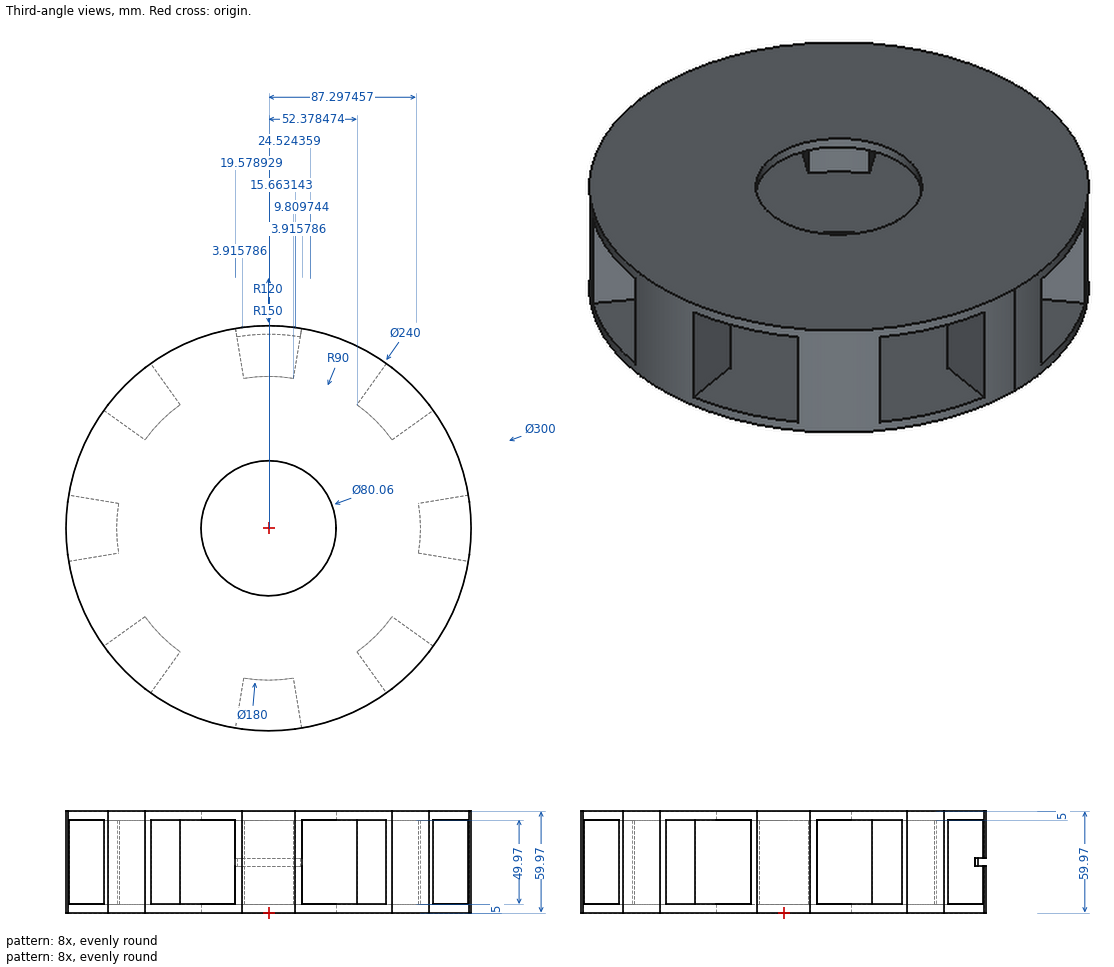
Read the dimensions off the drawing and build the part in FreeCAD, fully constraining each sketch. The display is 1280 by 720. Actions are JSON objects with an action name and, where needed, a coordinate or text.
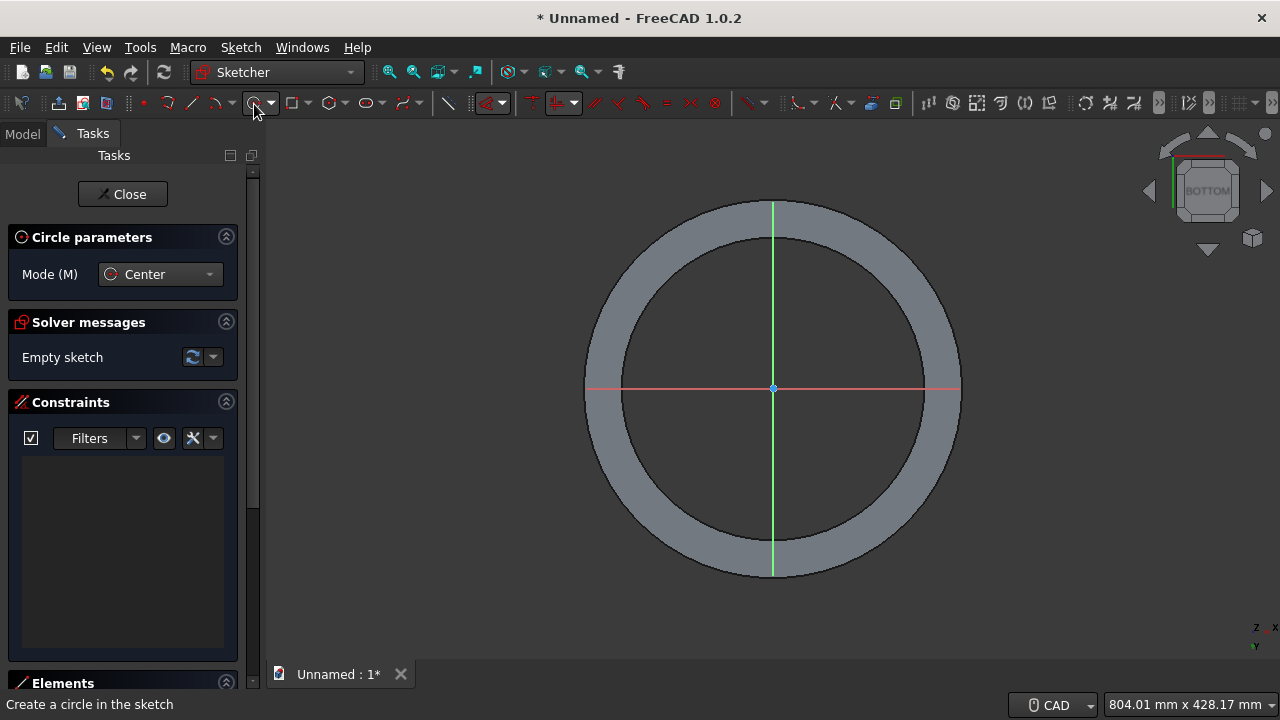
{"action": "left_click", "coordinate": [773, 389]}
{"action": "left_click", "coordinate": [880, 282]}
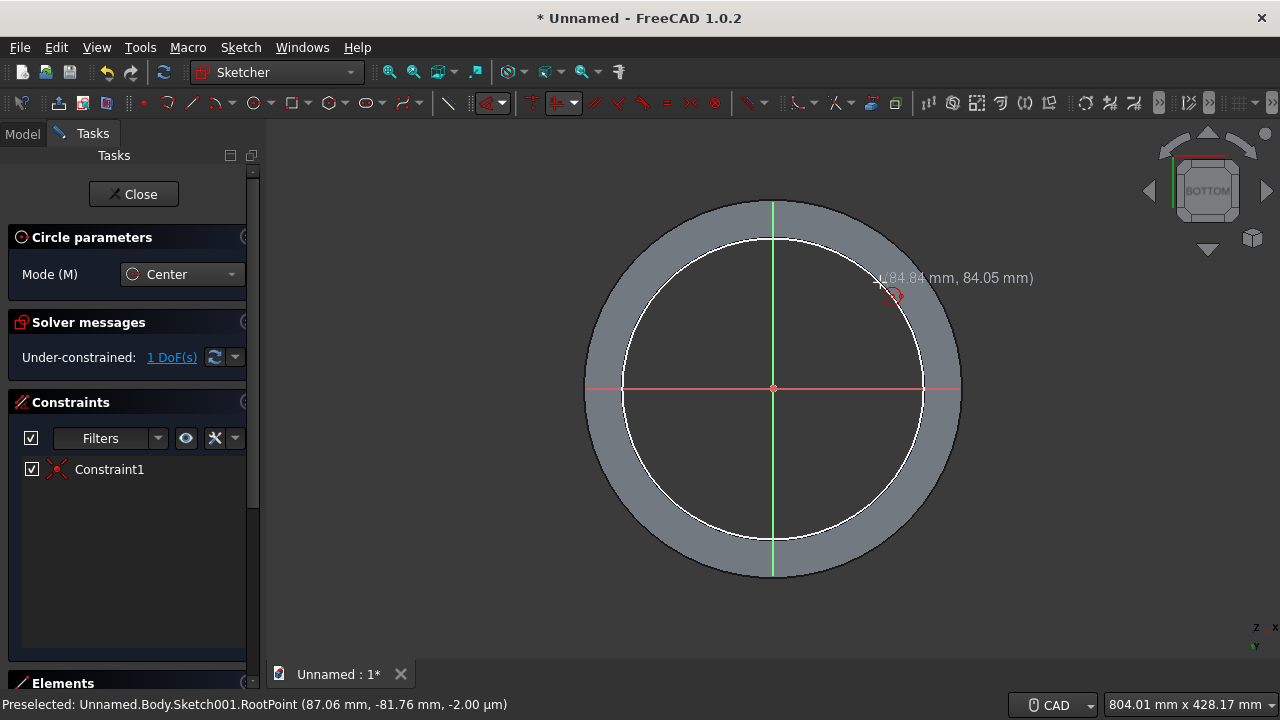
{"action": "left_click", "coordinate": [773, 389]}
{"action": "left_click", "coordinate": [853, 309]}
{"action": "key", "text": "Escape"}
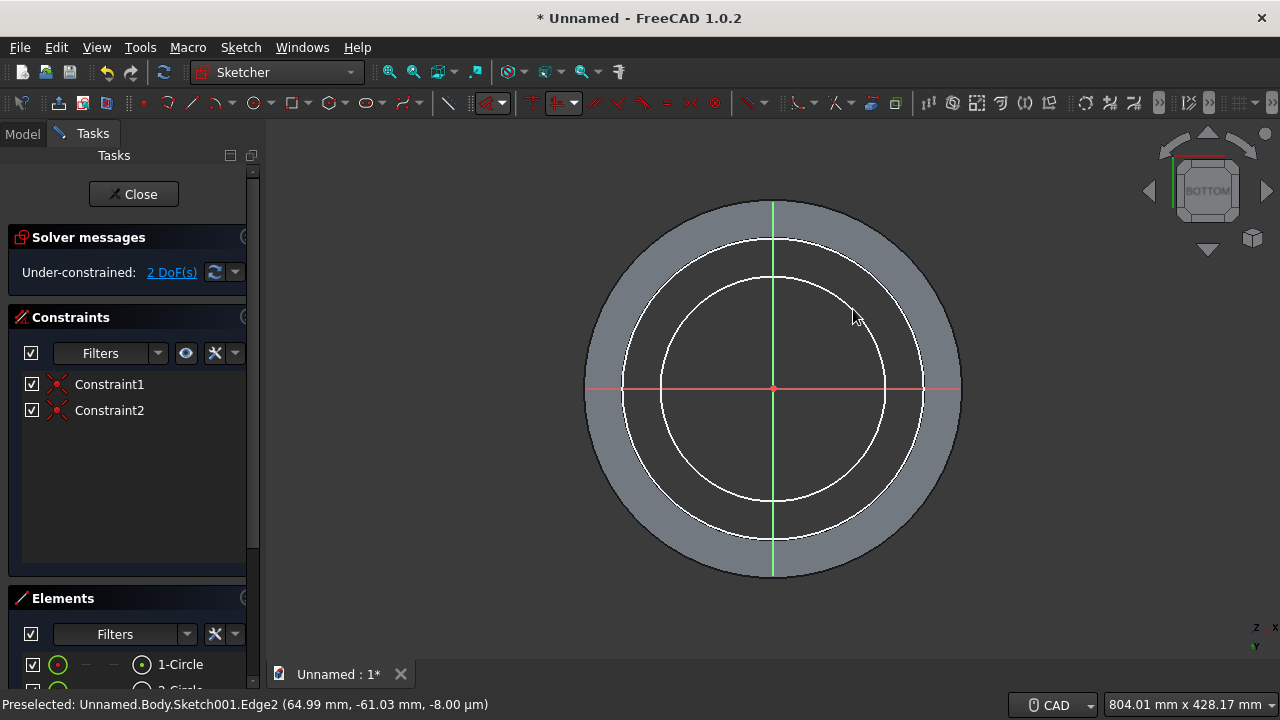
{"action": "left_click", "coordinate": [486, 104]}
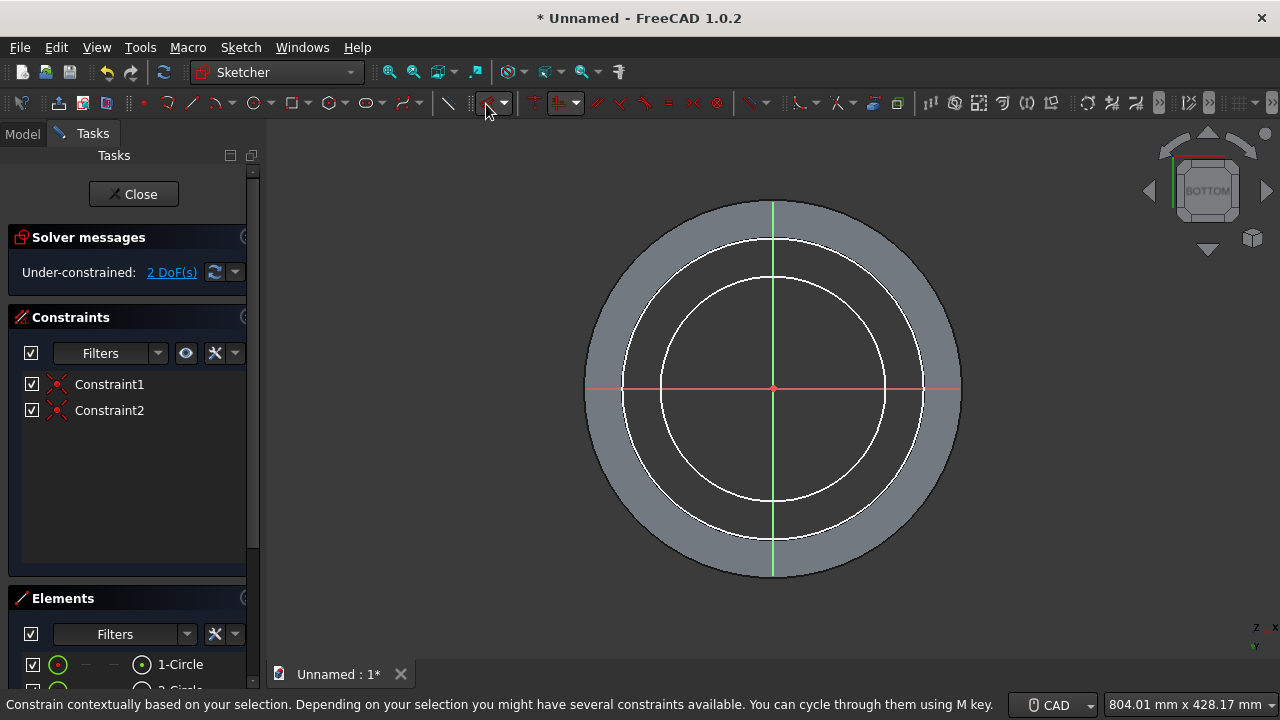
{"action": "left_click", "coordinate": [879, 282]}
{"action": "left_click", "coordinate": [902, 259]}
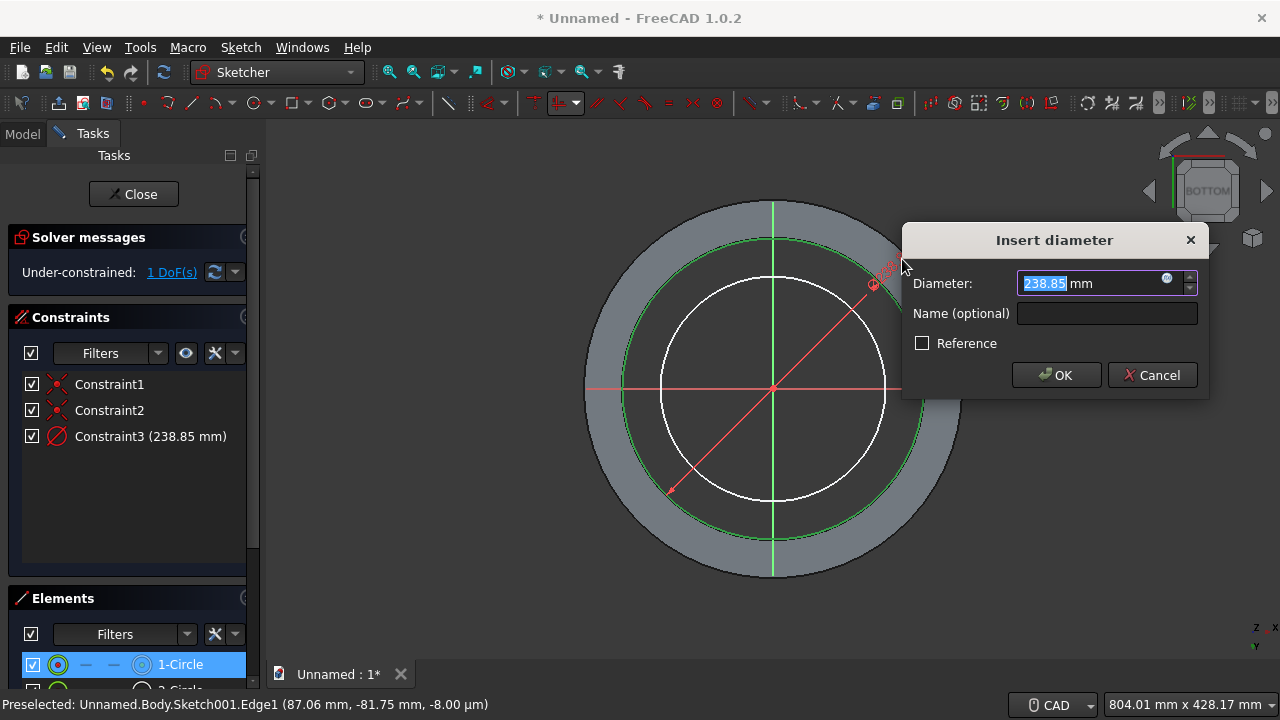
{"action": "type", "text": "240"}
{"action": "key", "text": "Return"}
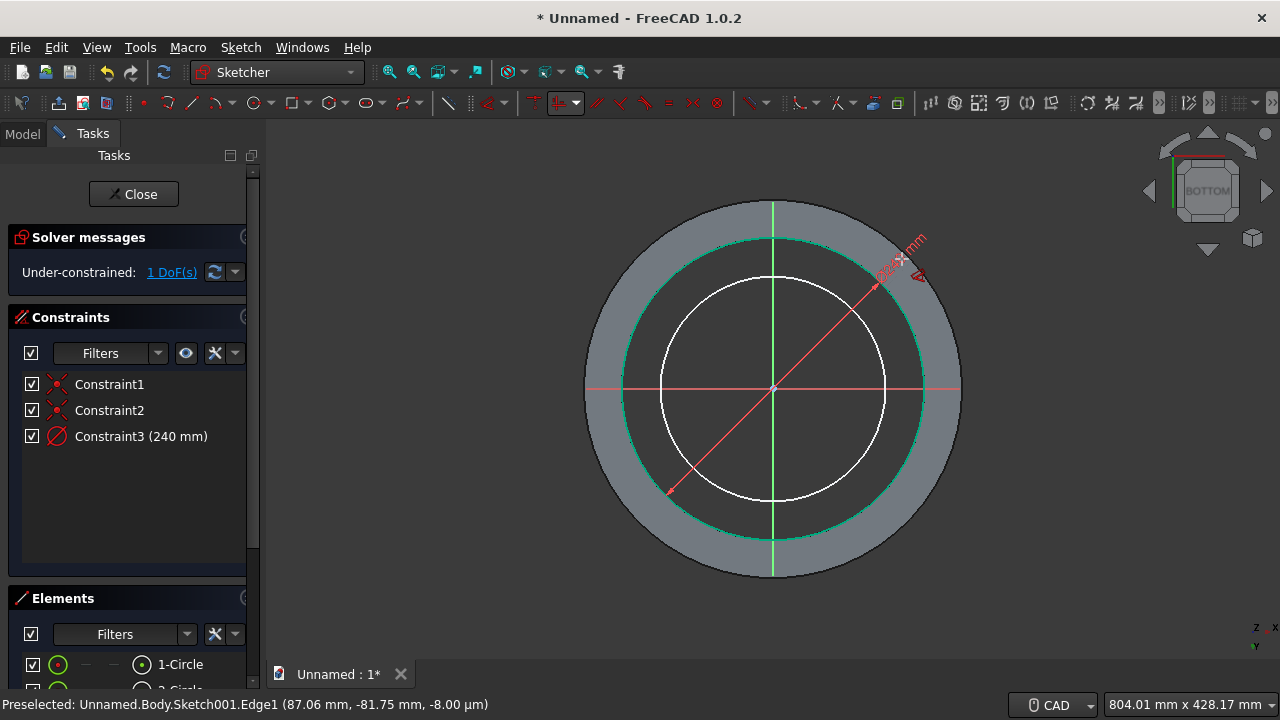
{"action": "left_click", "coordinate": [852, 309]}
{"action": "left_click", "coordinate": [933, 341]}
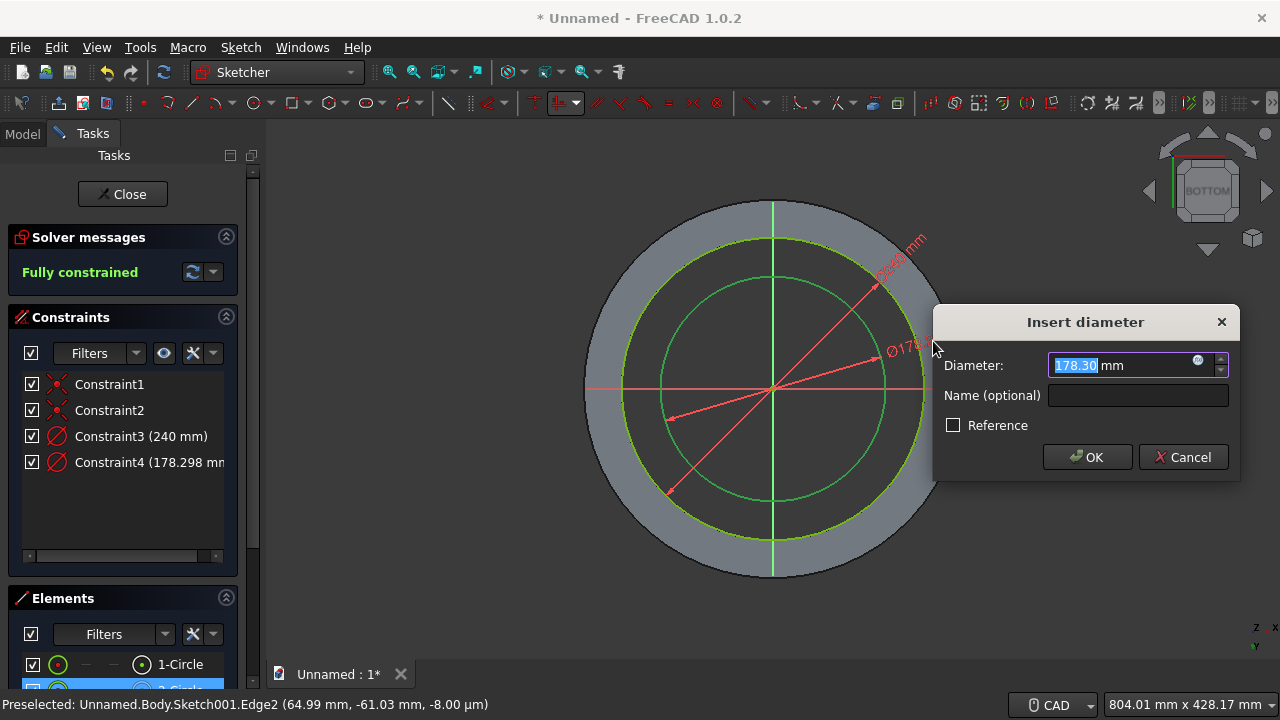
{"action": "type", "text": "180"}
{"action": "key", "text": "Return"}
{"action": "key", "text": "Escape"}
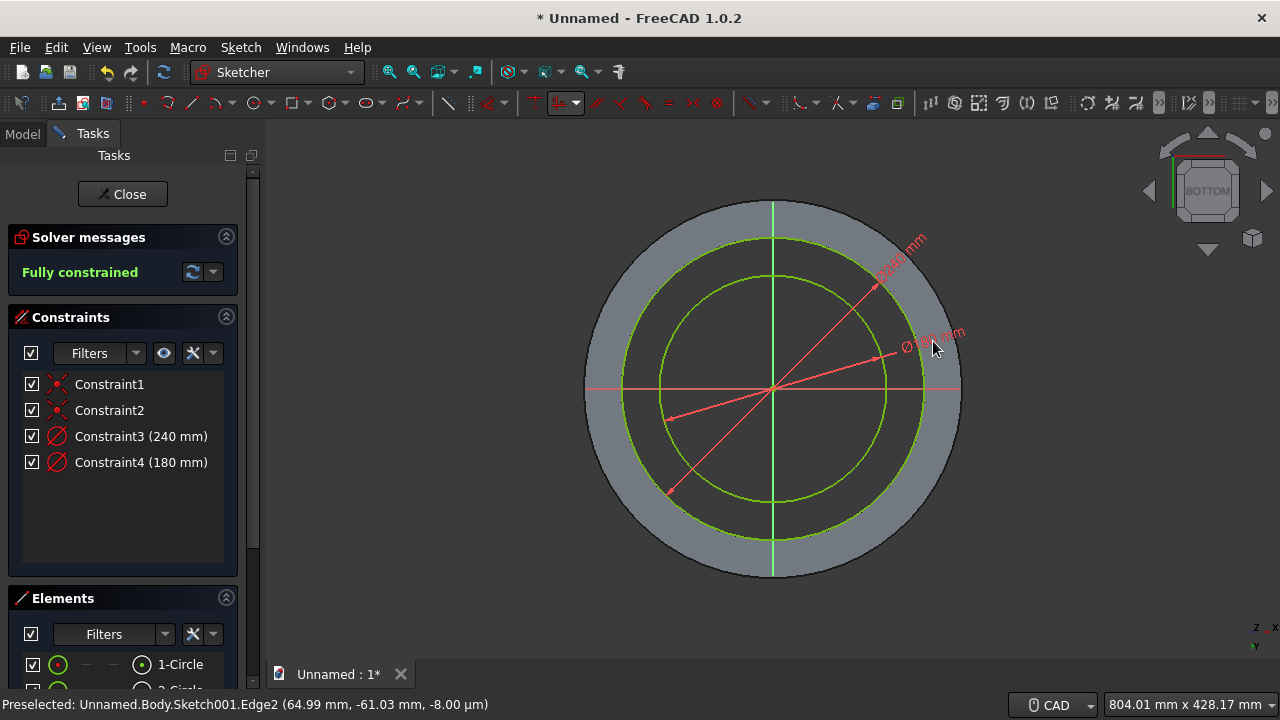
{"action": "left_click", "coordinate": [123, 194]}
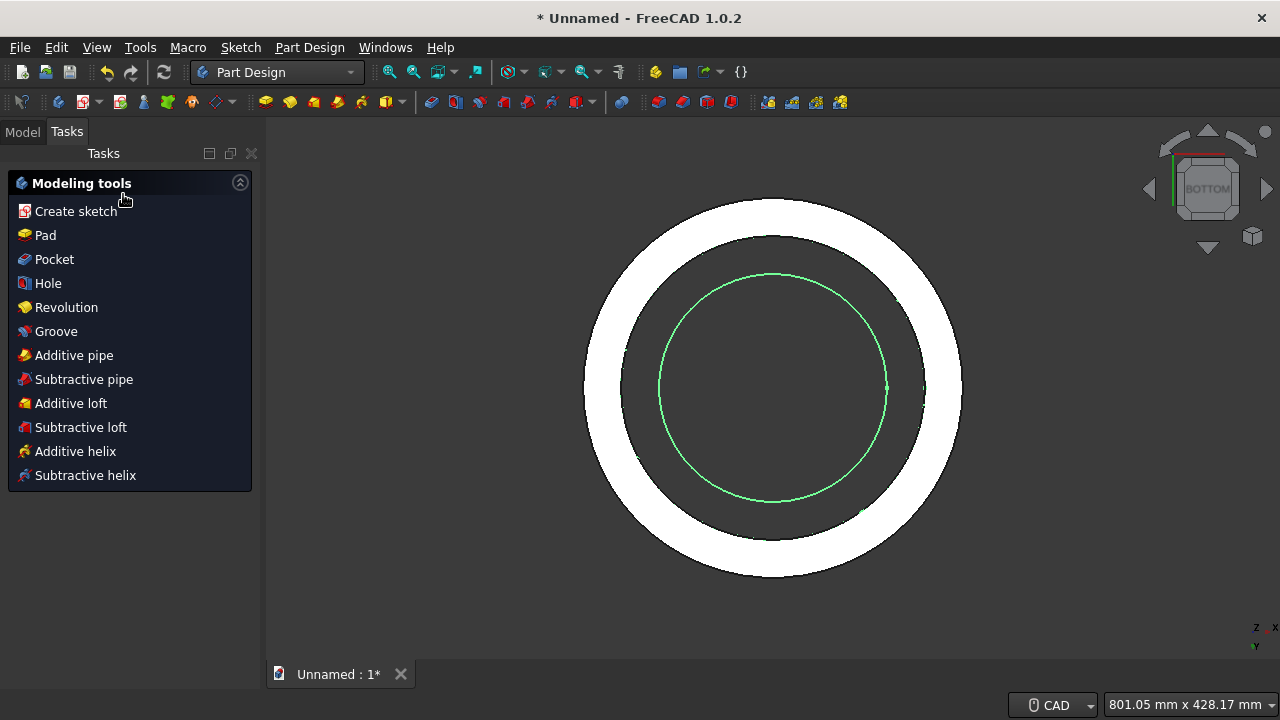
{"action": "left_click", "coordinate": [266, 102]}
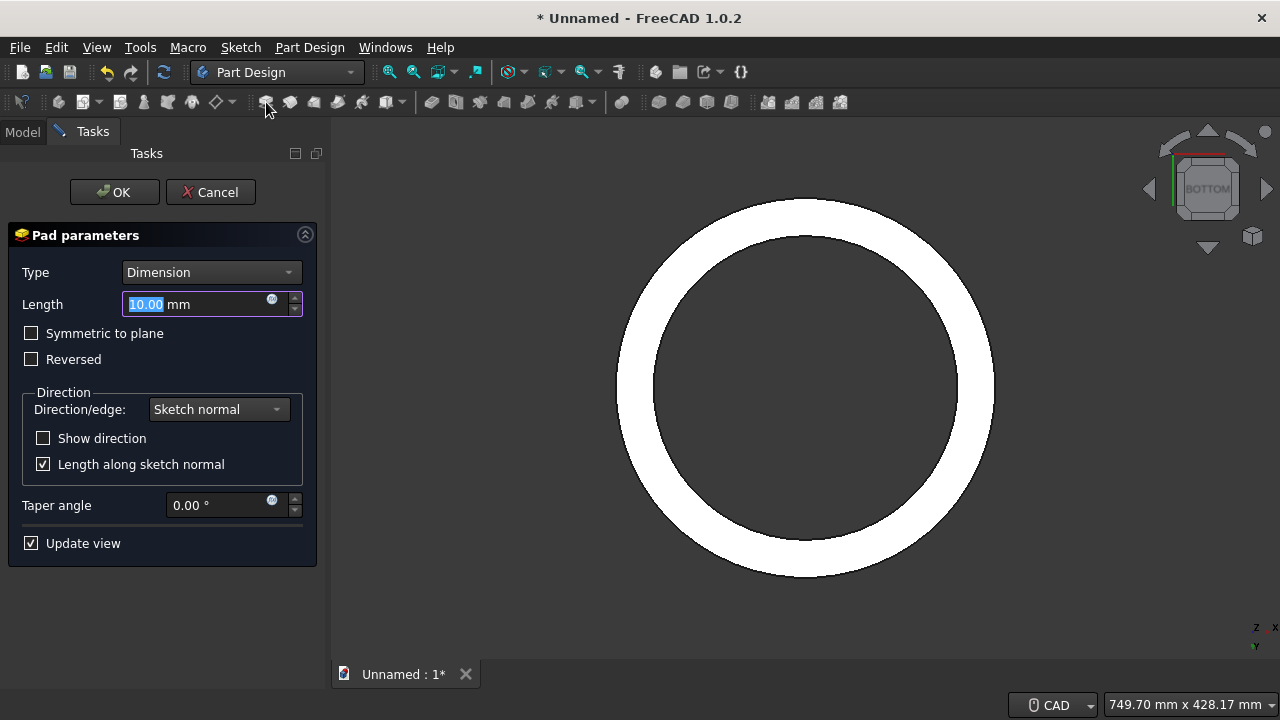
{"action": "type", "text": "59.97"}
{"action": "key", "text": "Tab"}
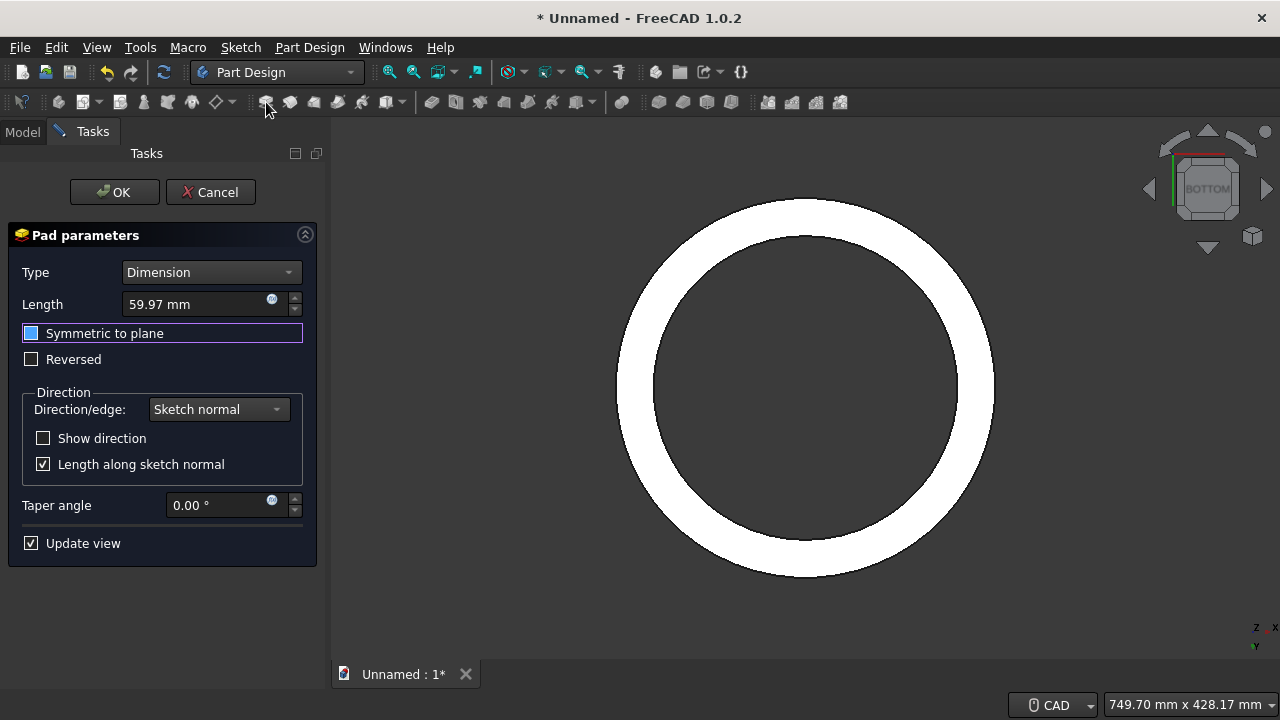
{"action": "left_click", "coordinate": [30, 359]}